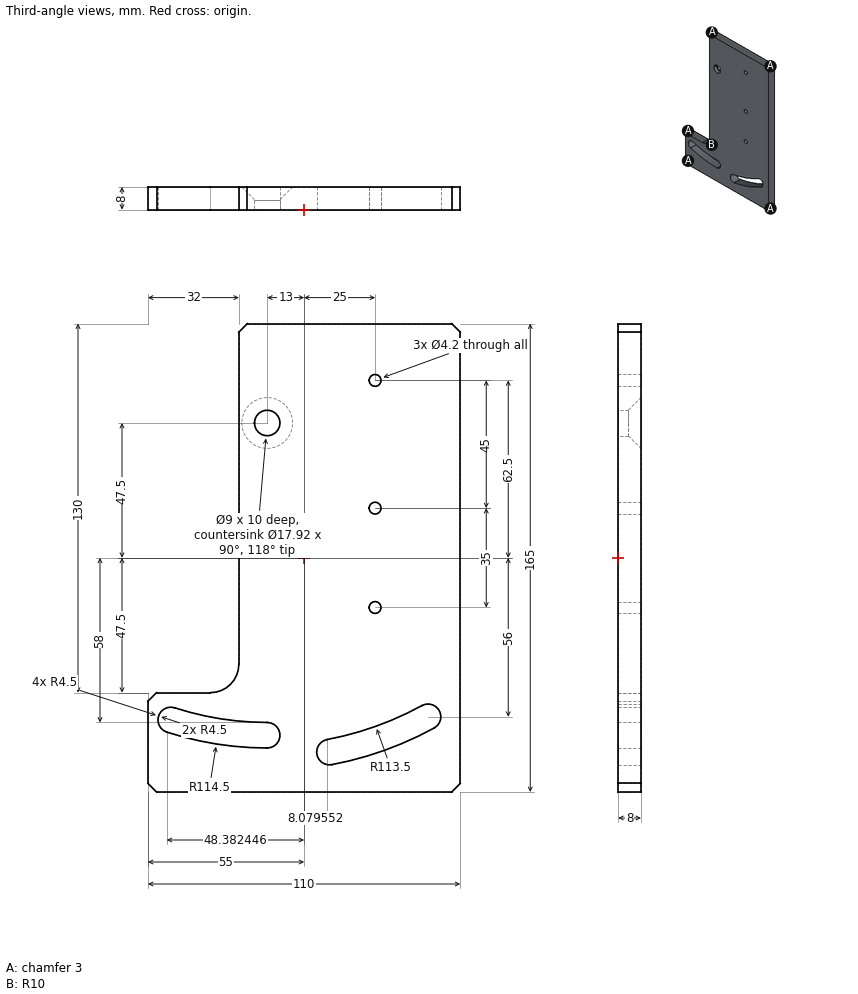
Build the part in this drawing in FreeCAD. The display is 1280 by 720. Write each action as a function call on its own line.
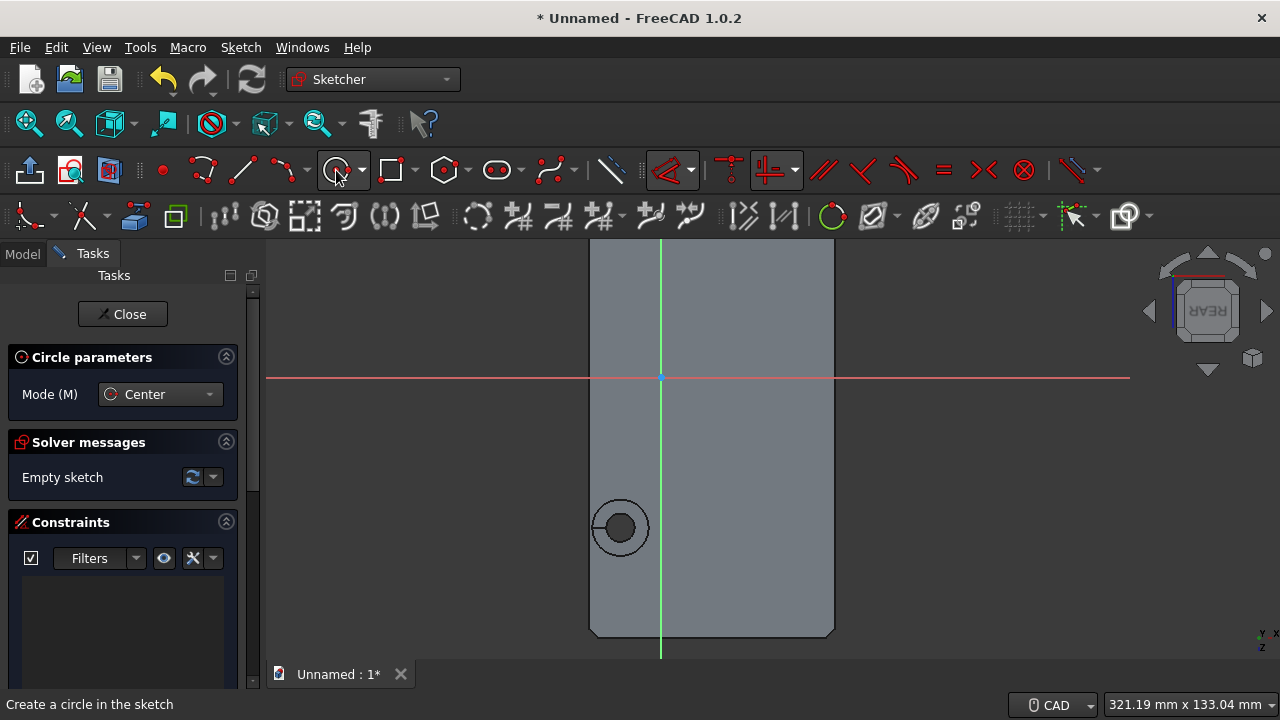
scroll(740, 575, up, 7)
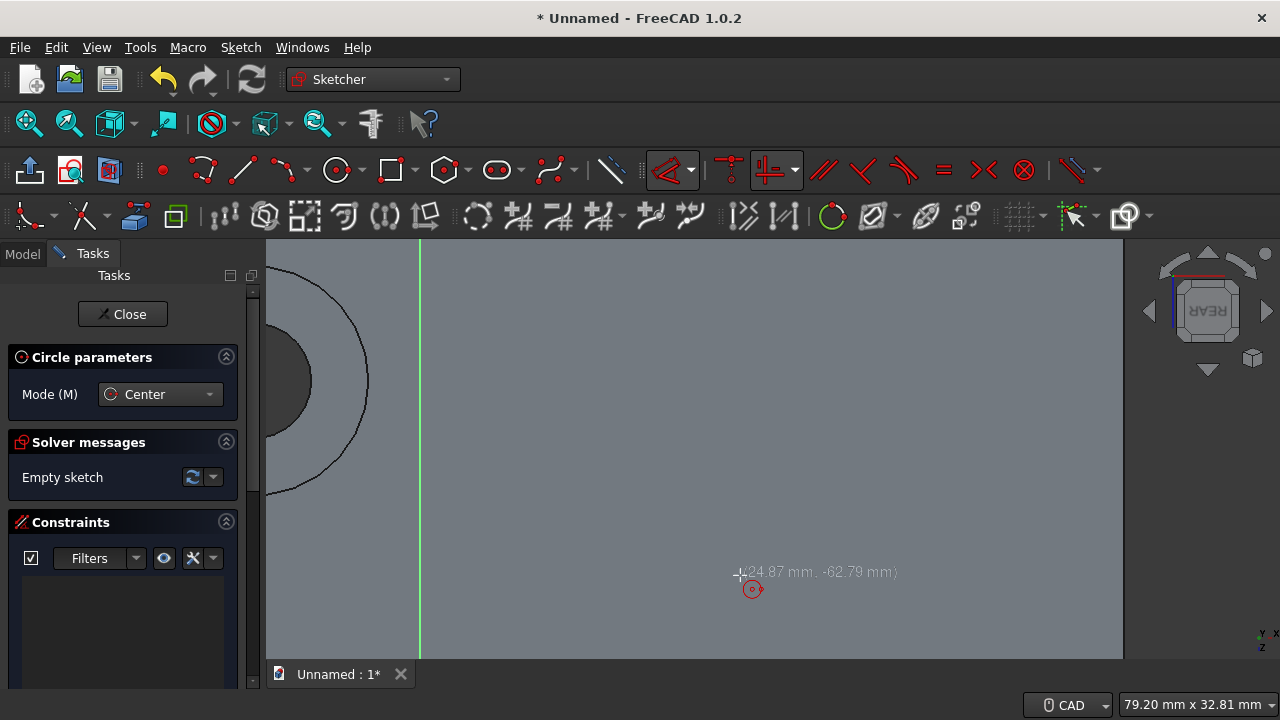
scroll(741, 576, down, 7)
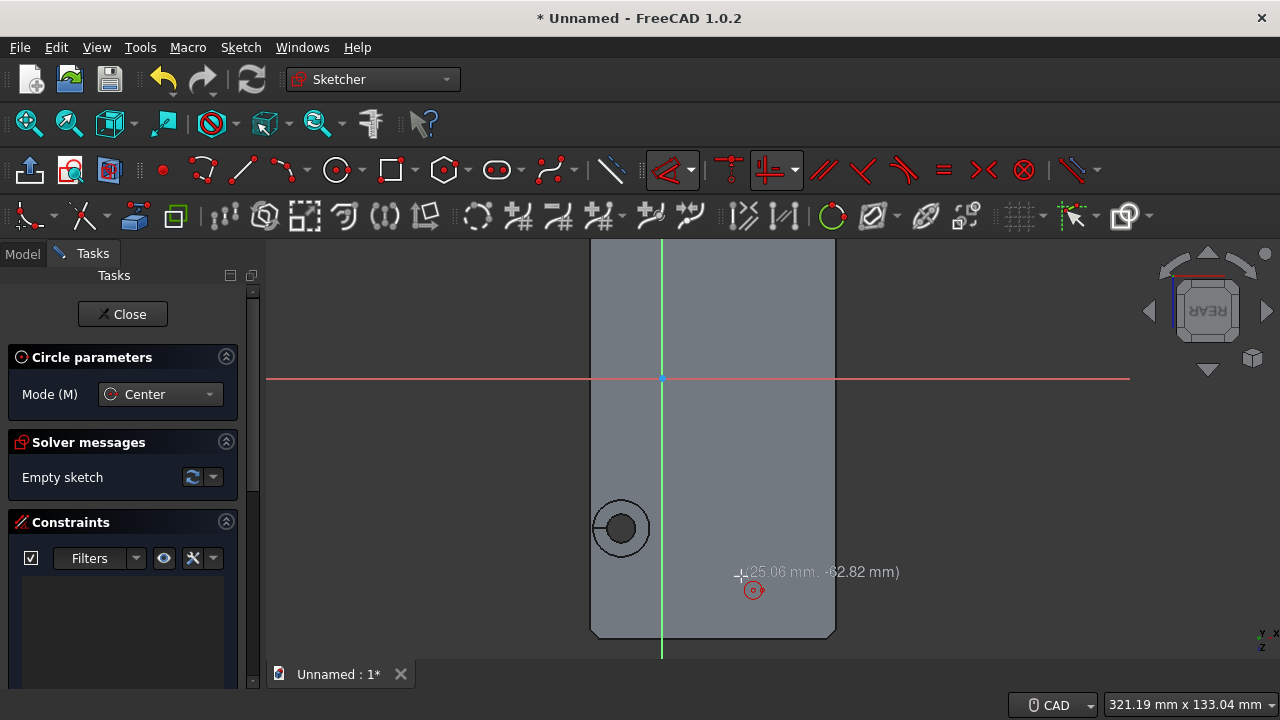
click(741, 576)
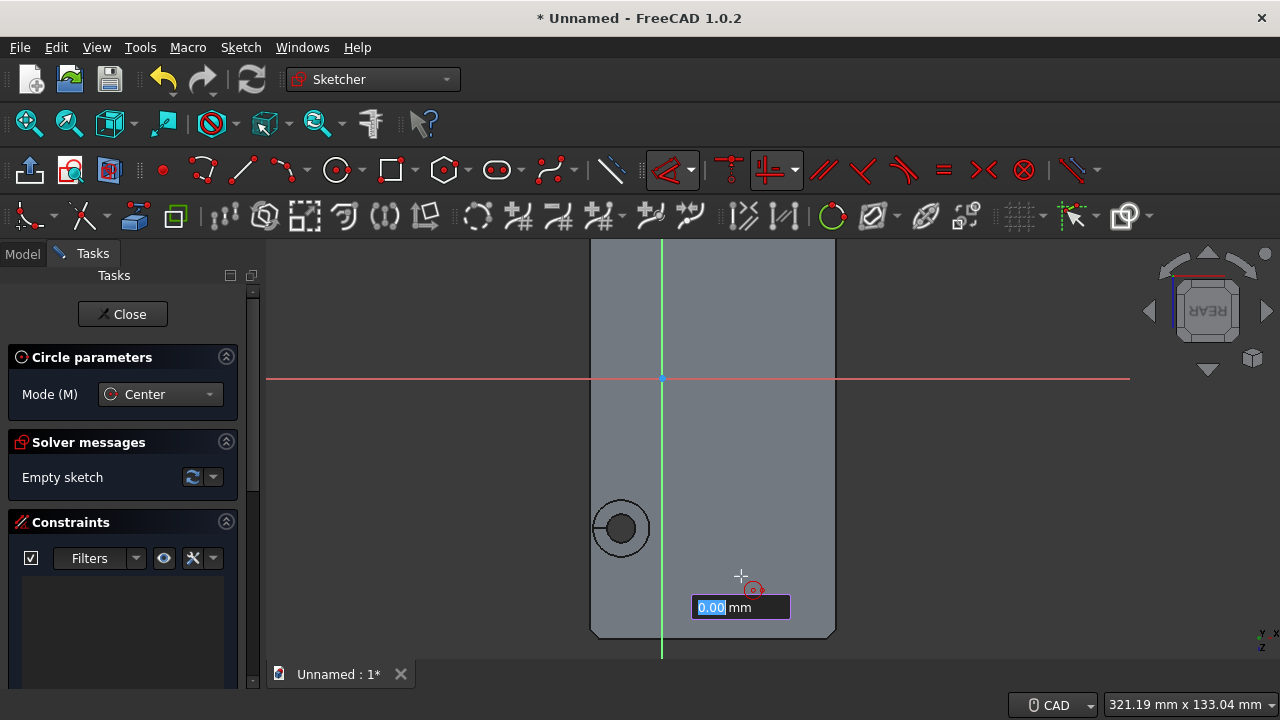
scroll(746, 571, up, 5)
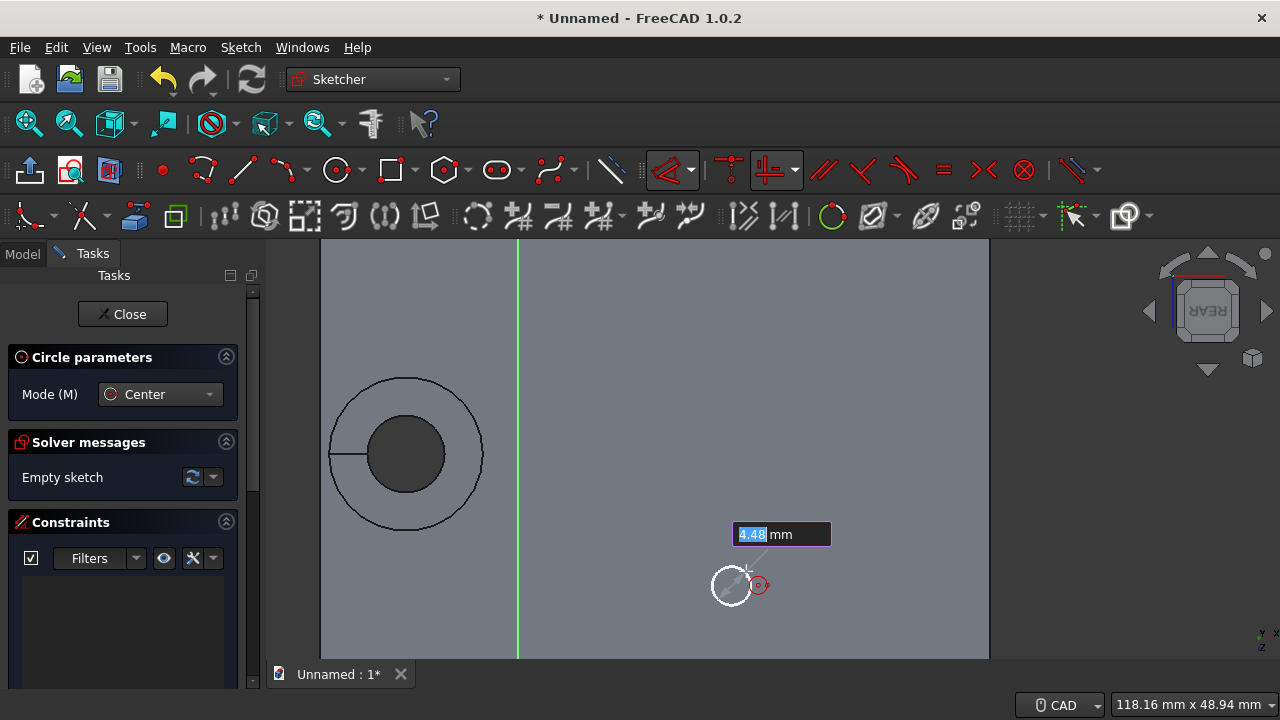
click(745, 570)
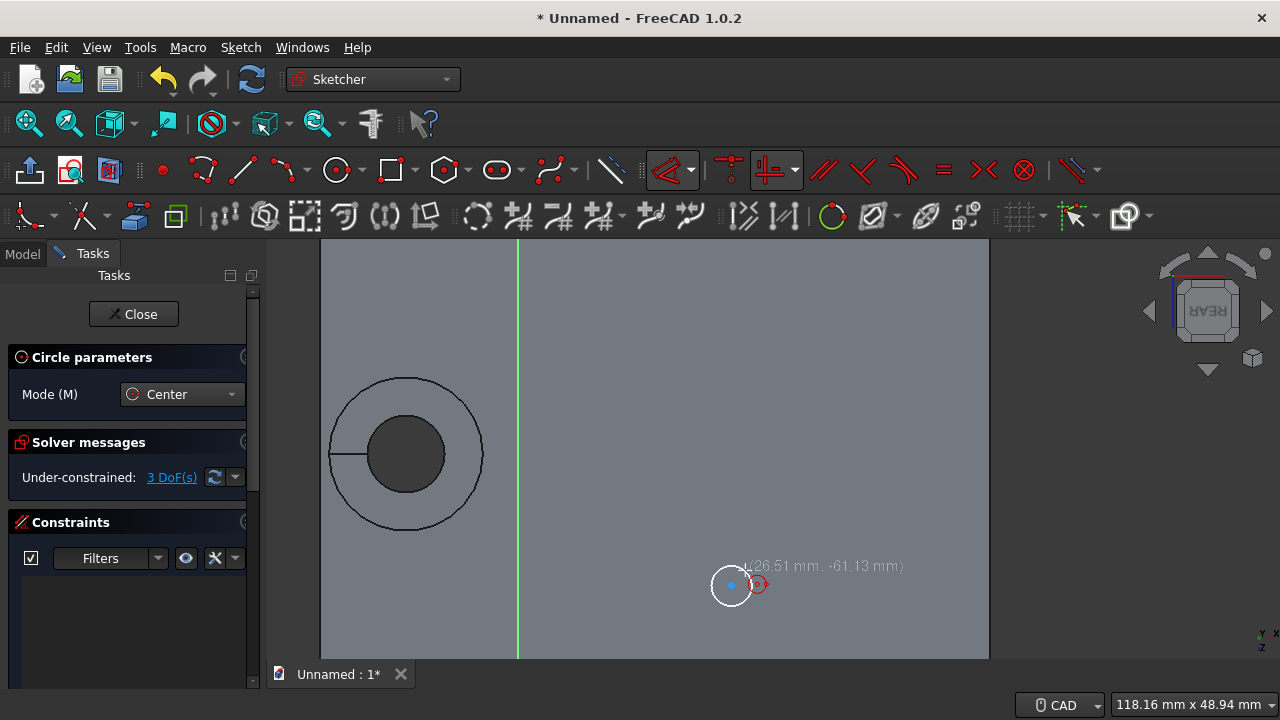
scroll(746, 571, down, 5)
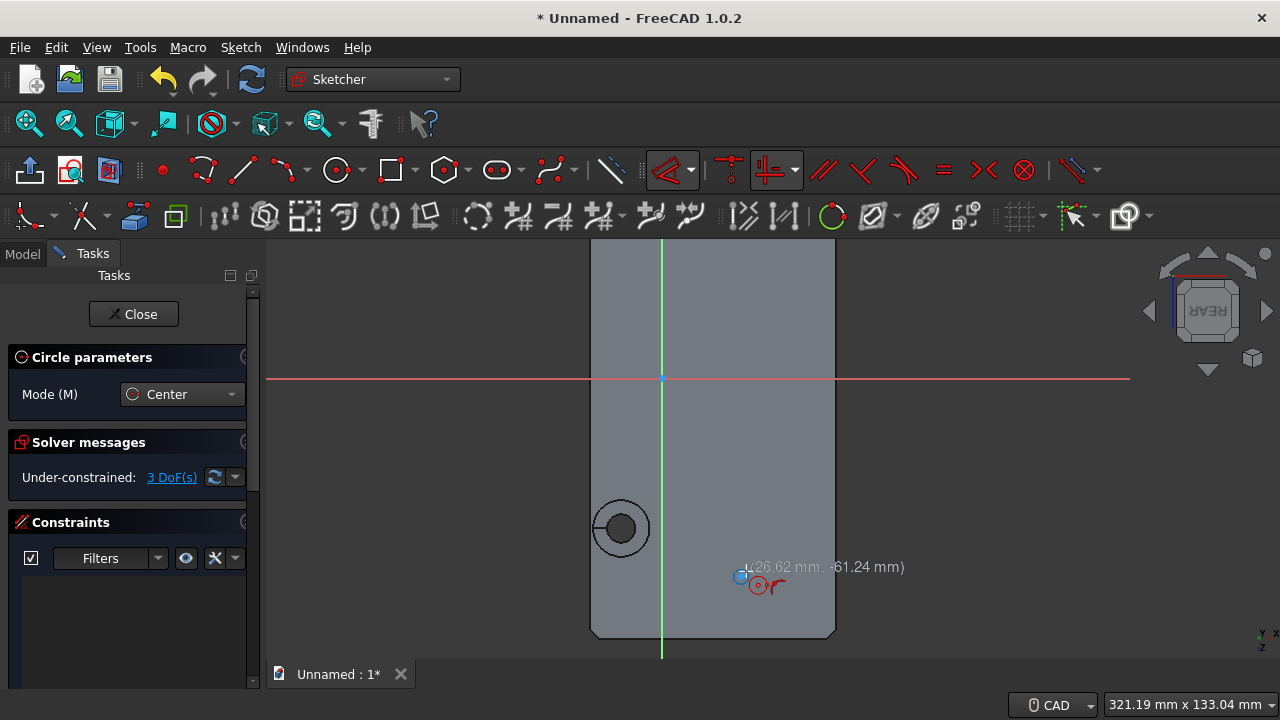
scroll(741, 434, up, 7)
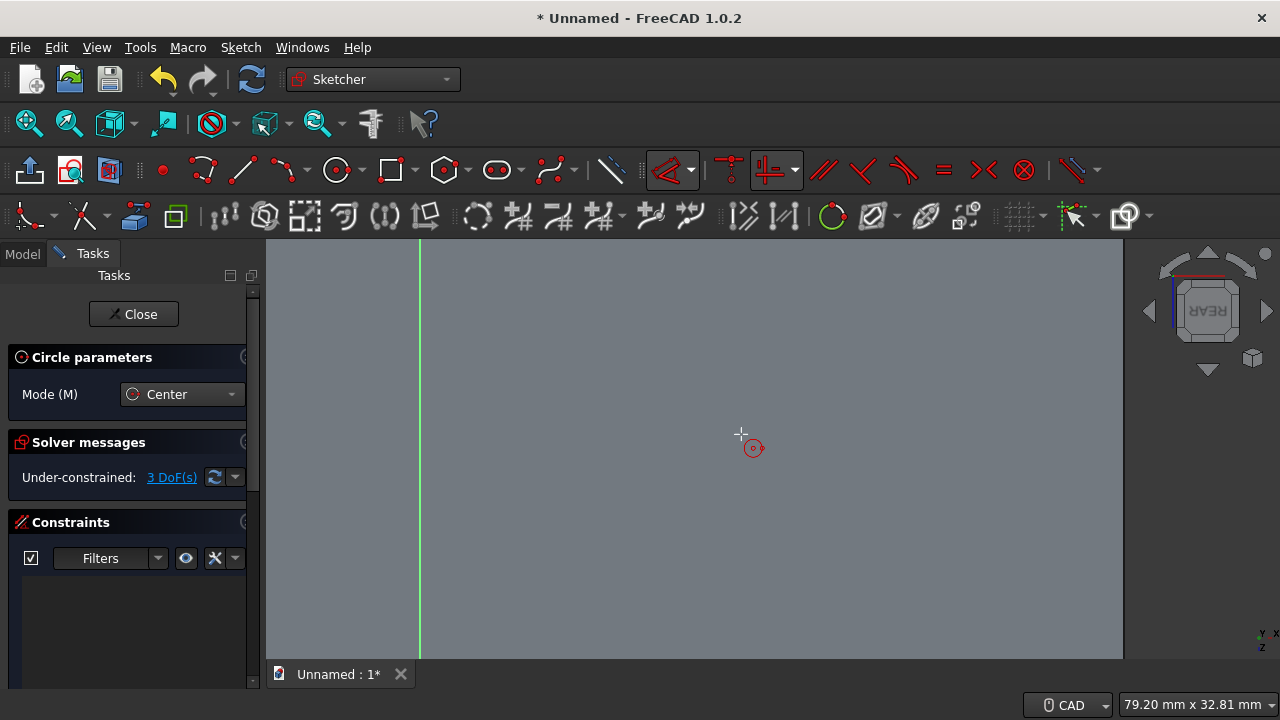
scroll(741, 434, down, 7)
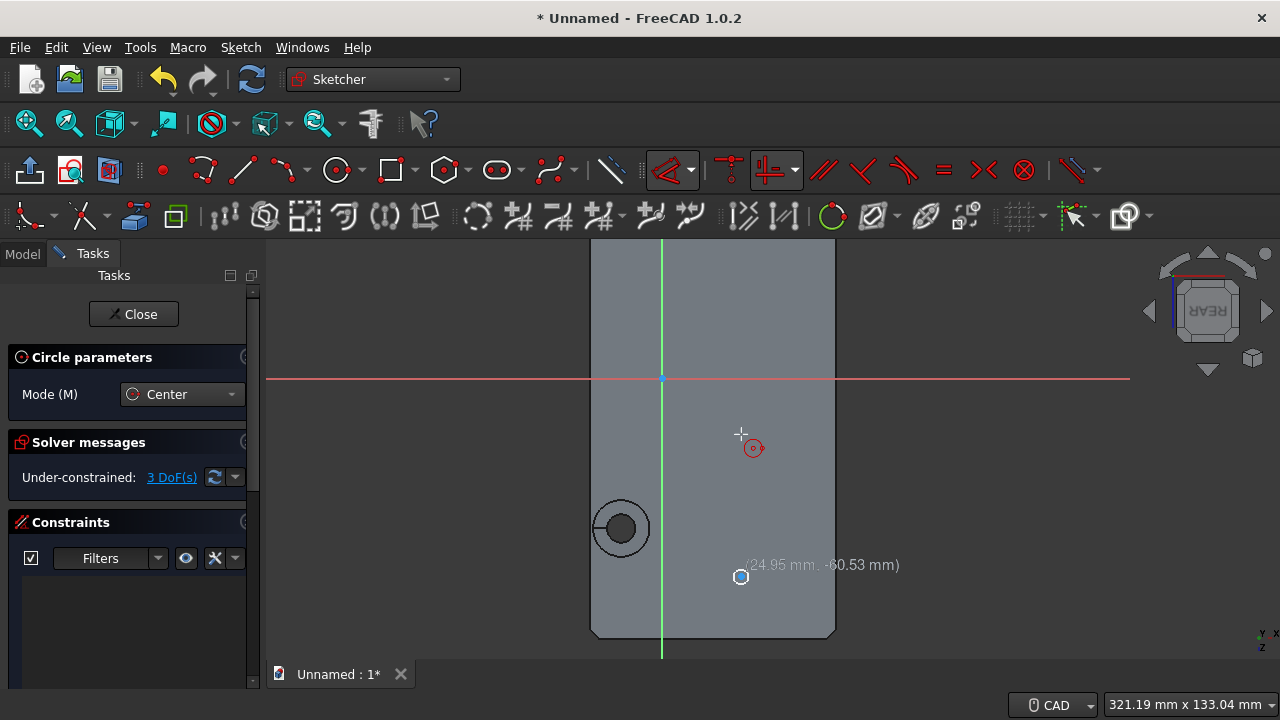
click(741, 434)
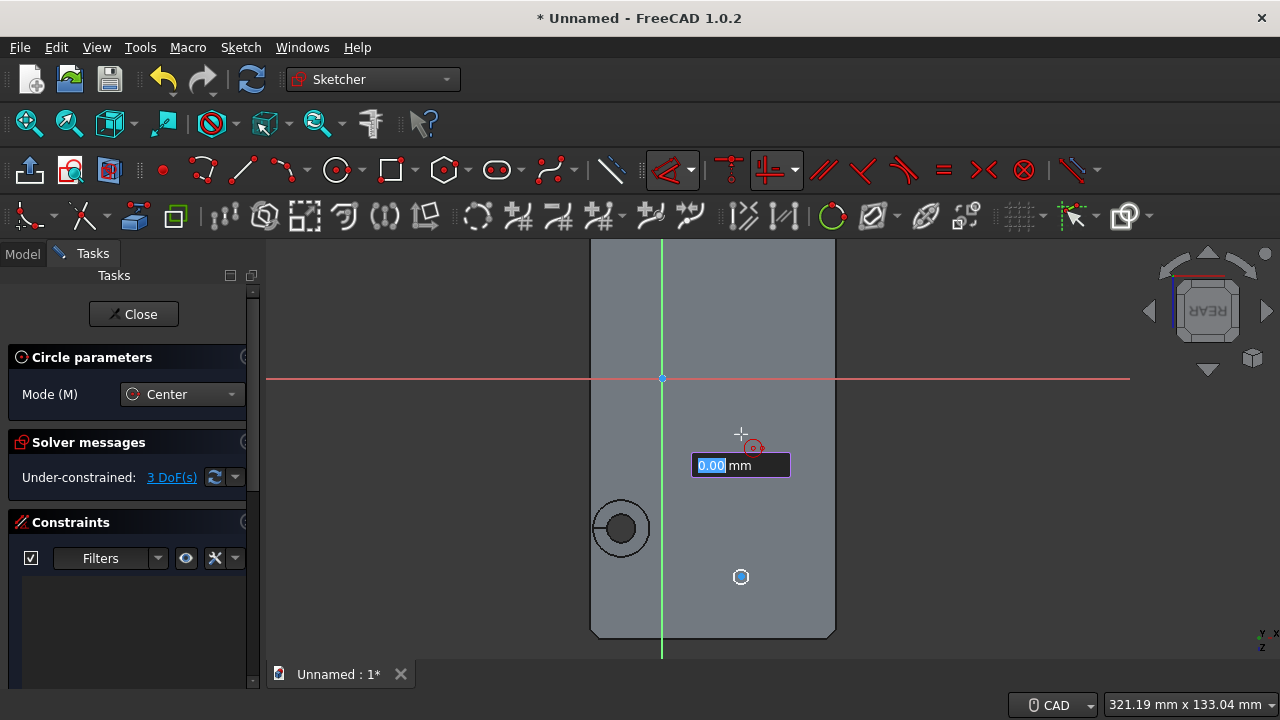
scroll(746, 429, up, 5)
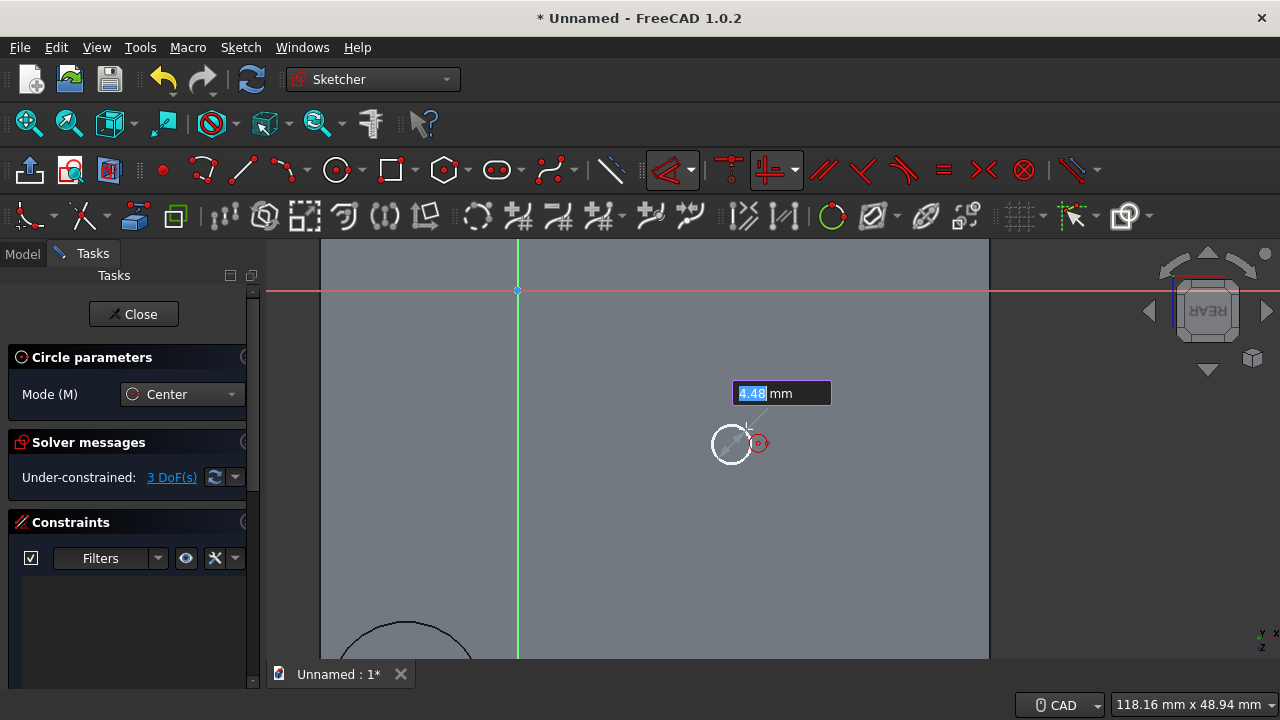
click(745, 428)